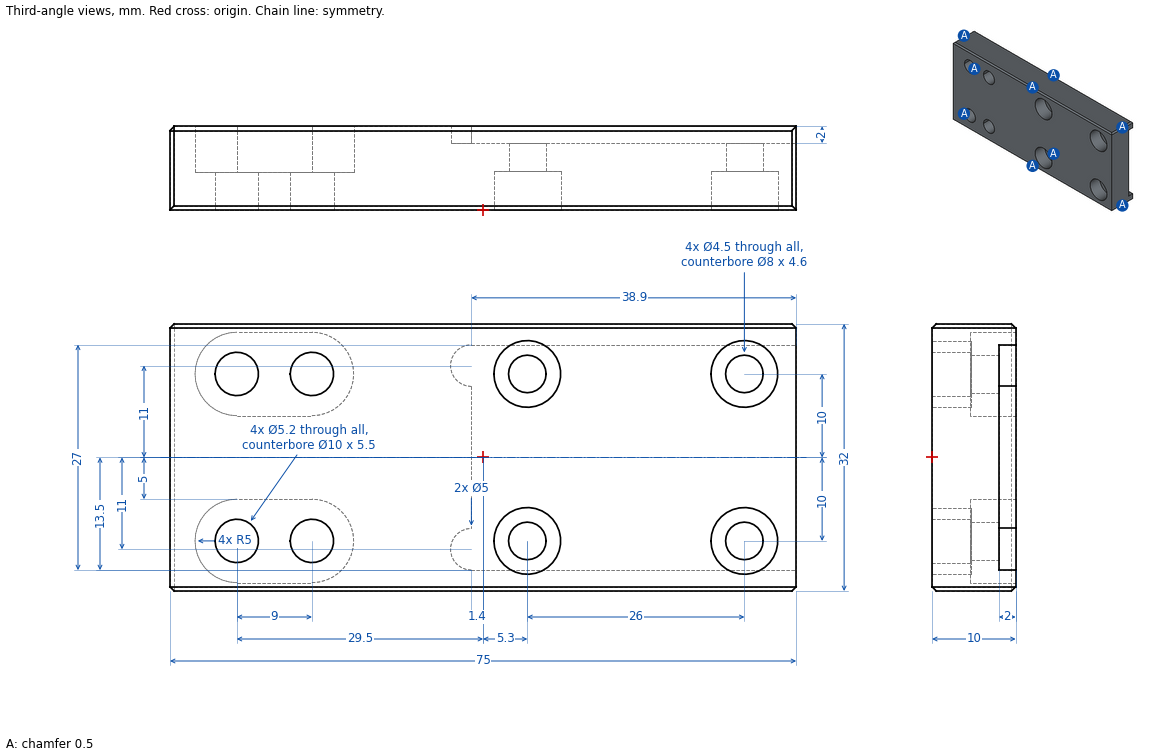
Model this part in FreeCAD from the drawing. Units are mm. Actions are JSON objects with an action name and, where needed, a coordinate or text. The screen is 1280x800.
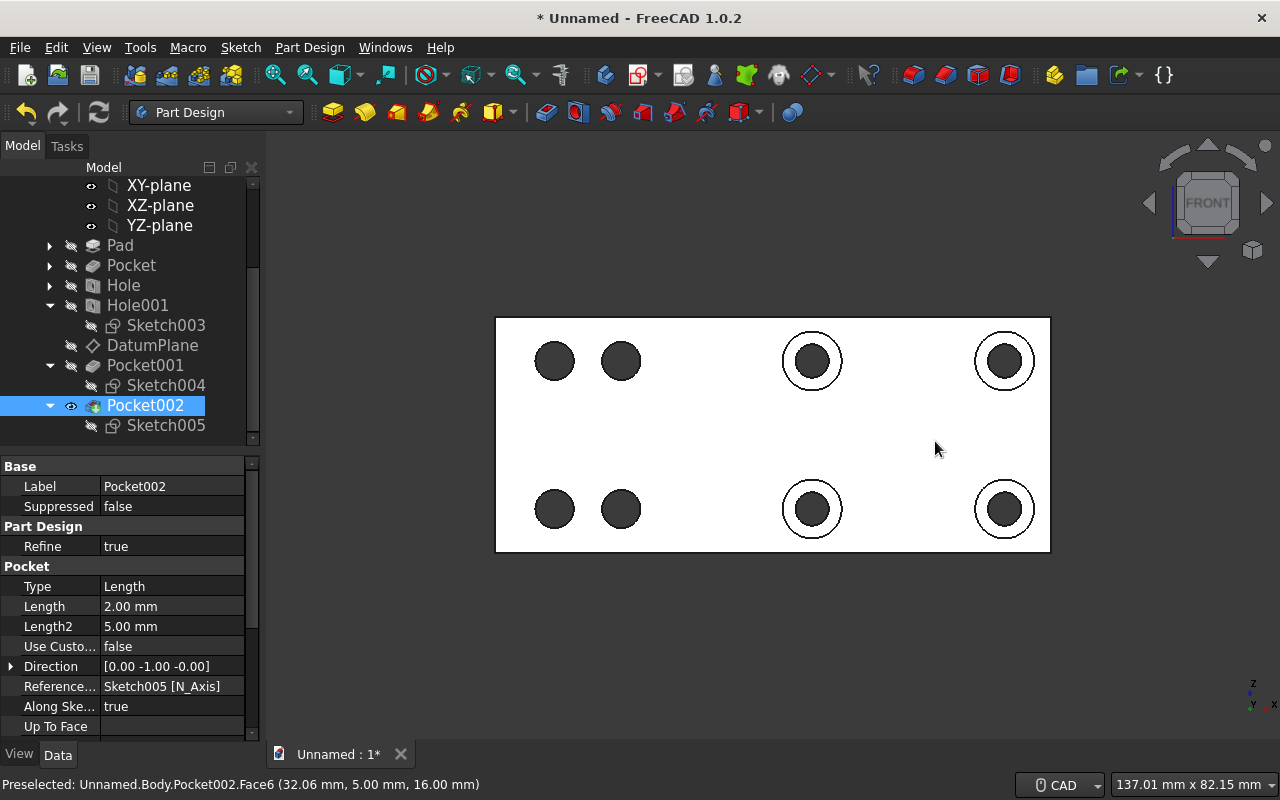
{"action": "key", "text": "3"}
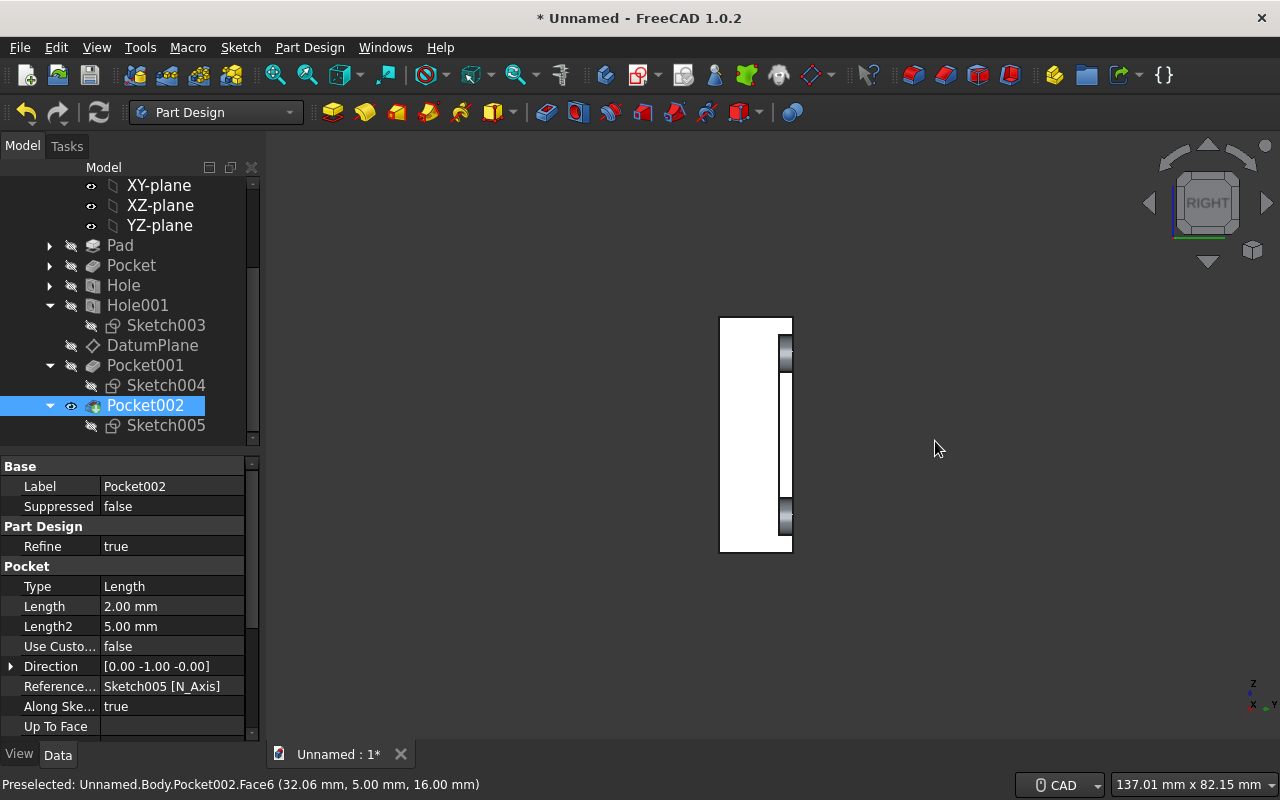
{"action": "left_click", "coordinate": [276, 76]}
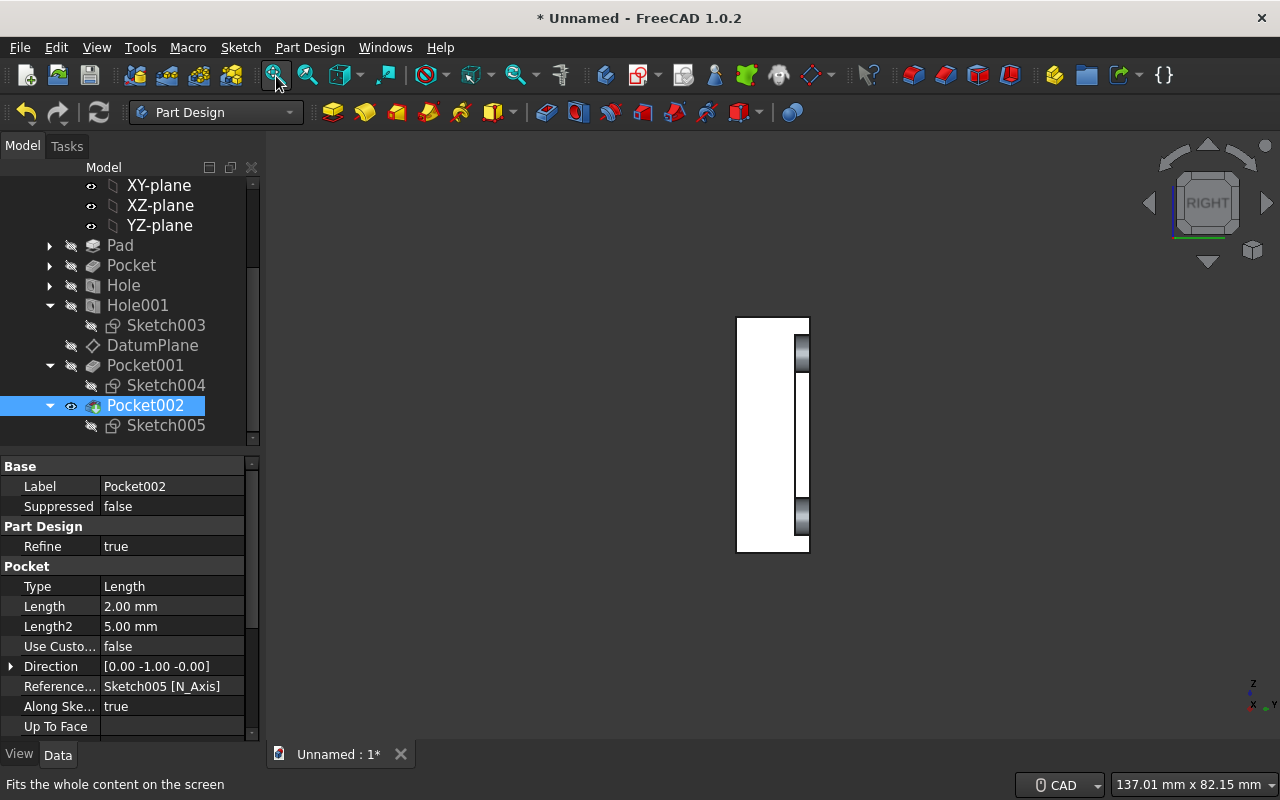
{"action": "key", "text": "5"}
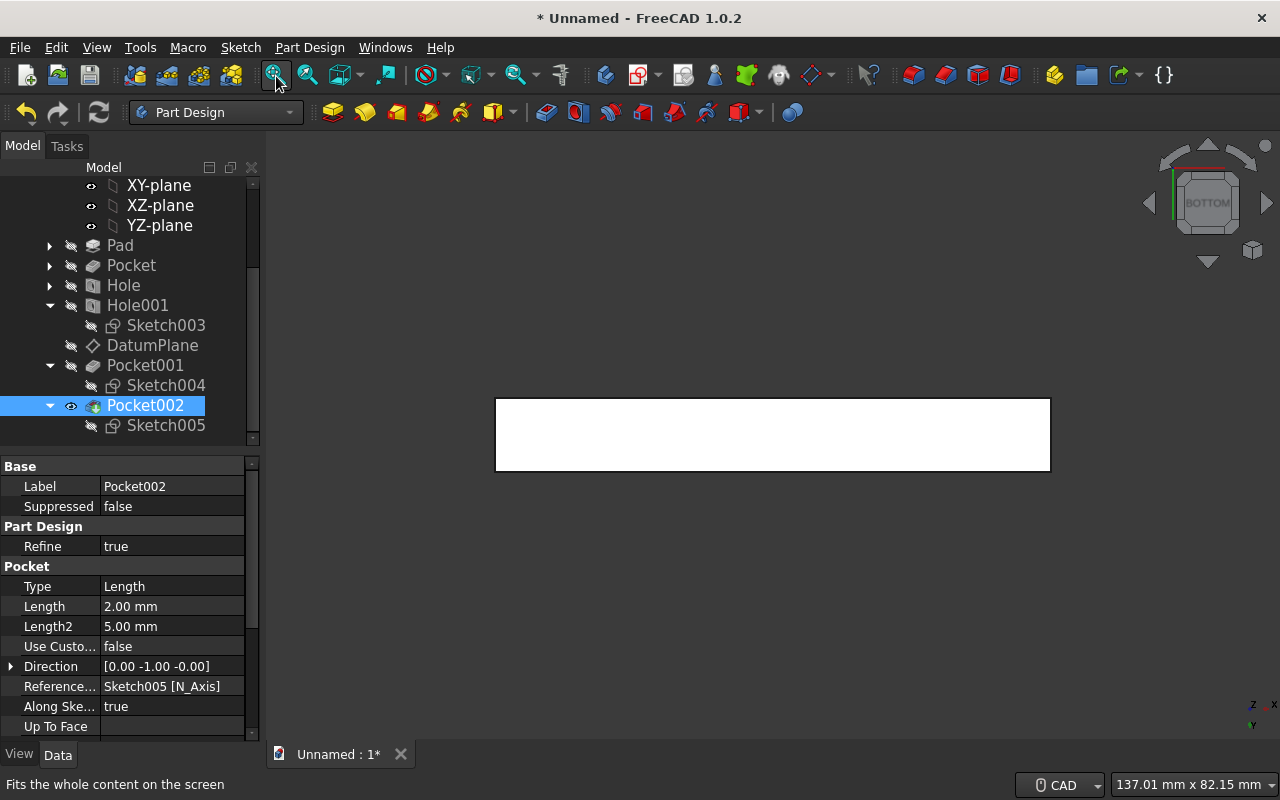
{"action": "left_click", "coordinate": [1011, 434], "text": "ctrl"}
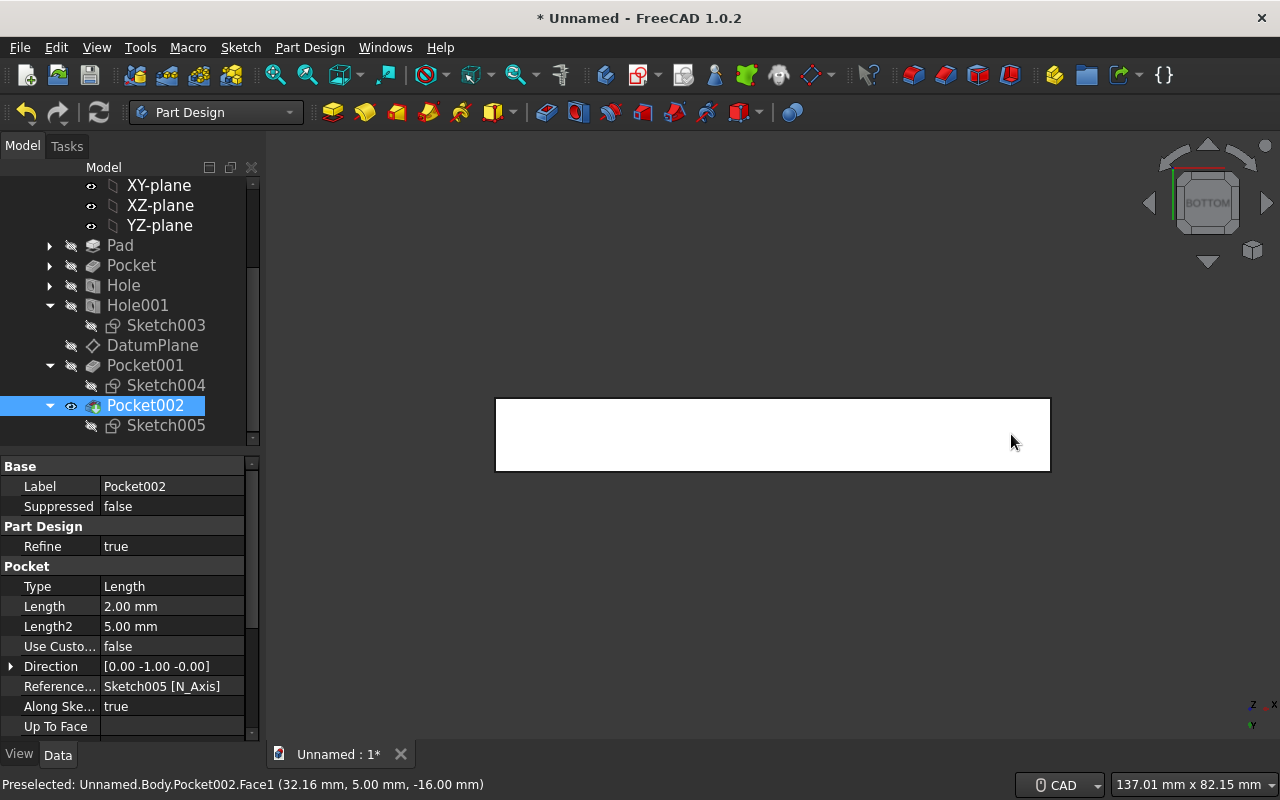
{"action": "left_click", "coordinate": [946, 76]}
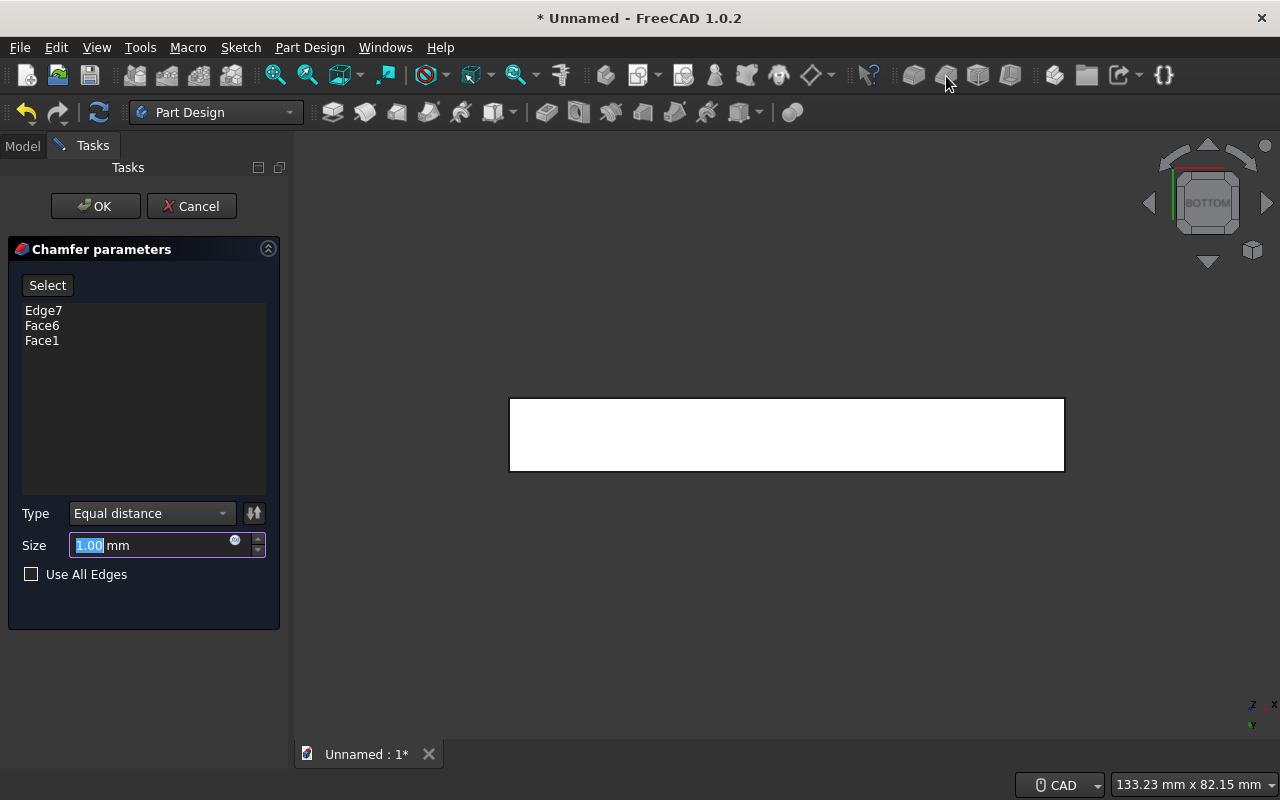
{"action": "type", "text": "0.5"}
{"action": "key", "text": "Tab"}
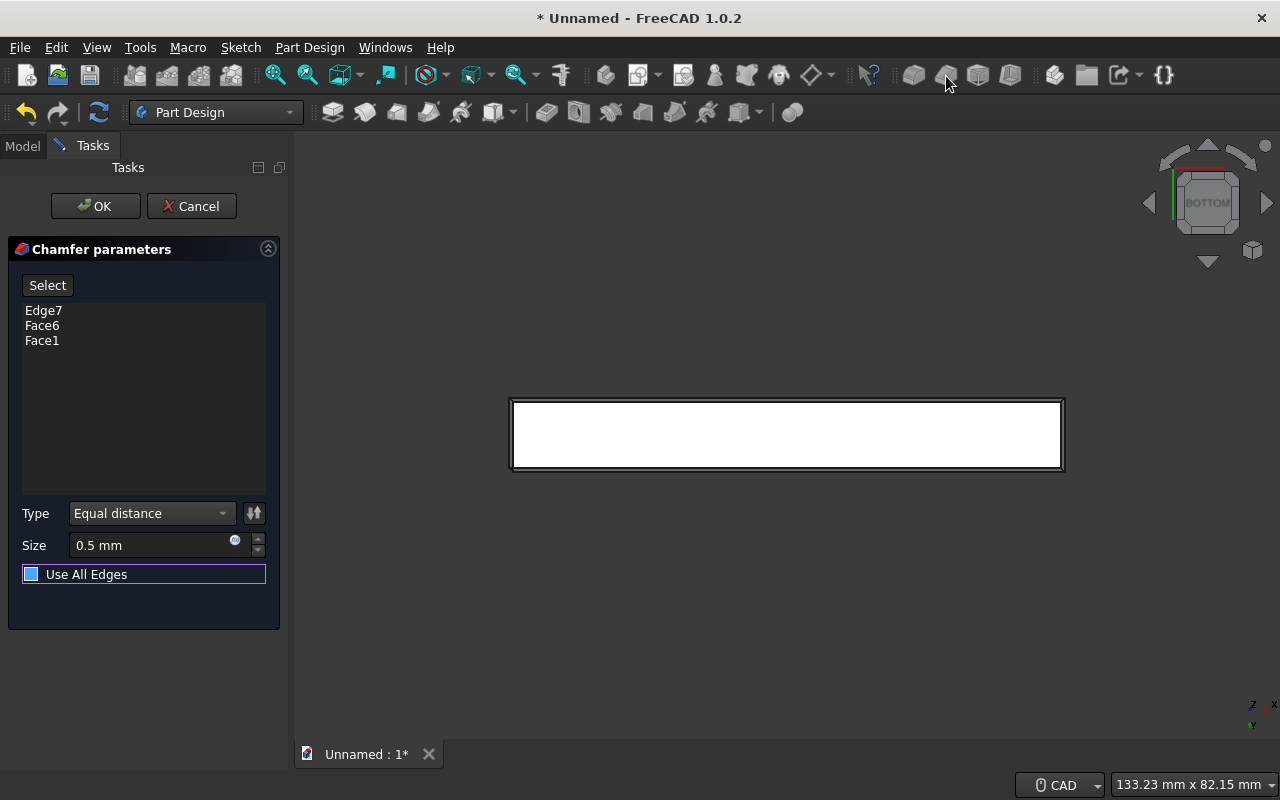
{"action": "left_click", "coordinate": [96, 206]}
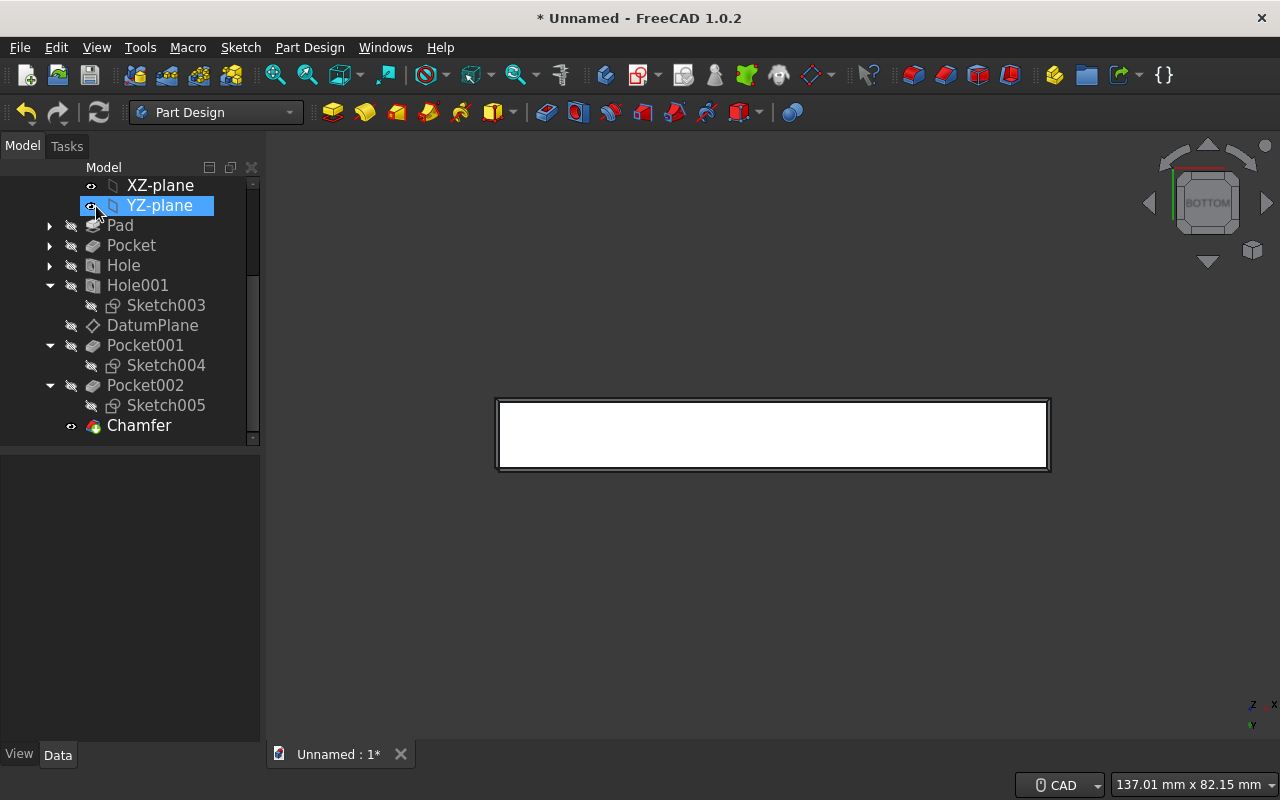
{"action": "key", "text": "0"}